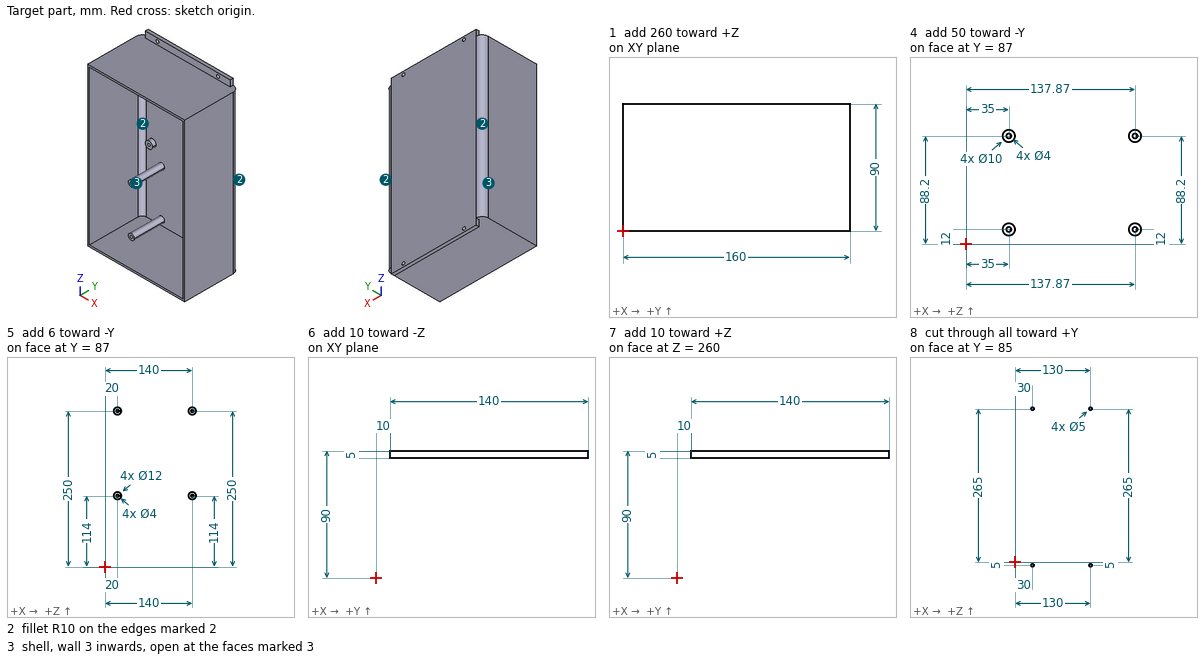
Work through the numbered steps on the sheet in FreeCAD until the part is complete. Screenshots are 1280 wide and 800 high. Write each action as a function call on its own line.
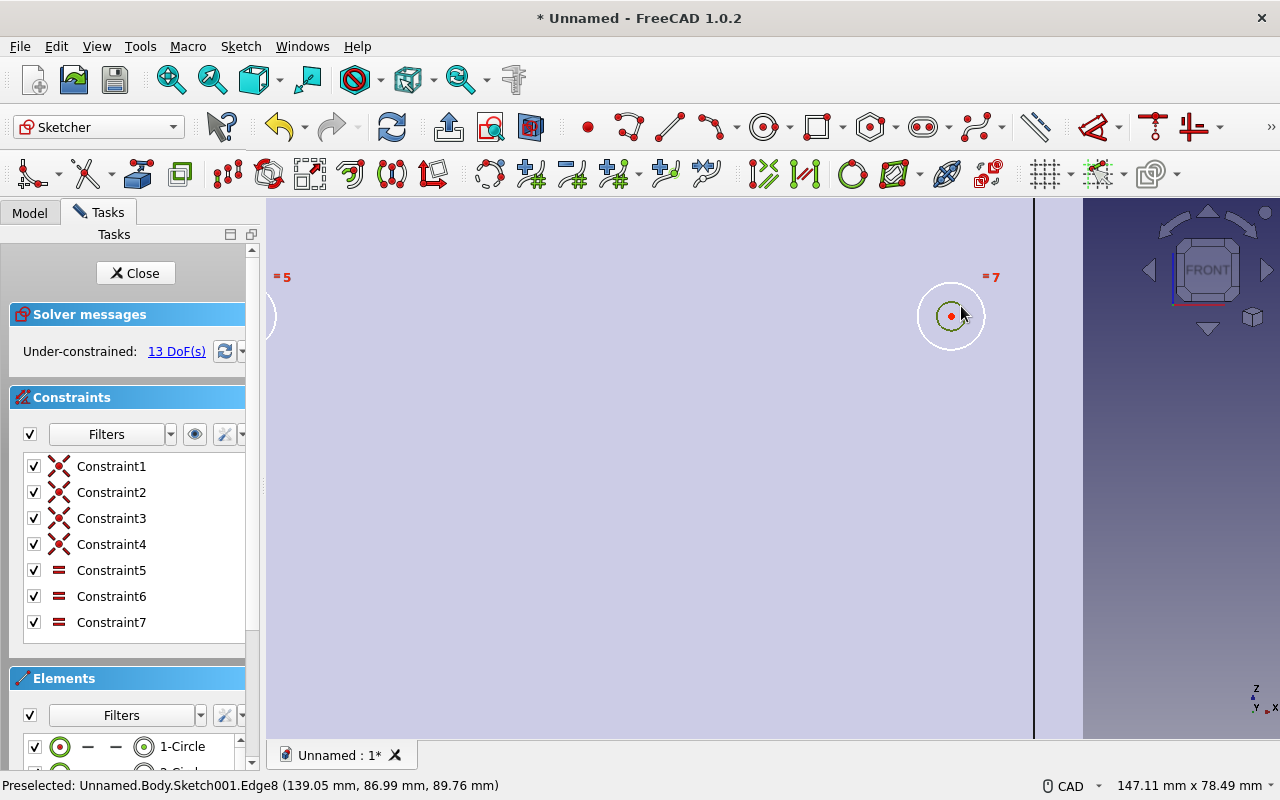
key(e)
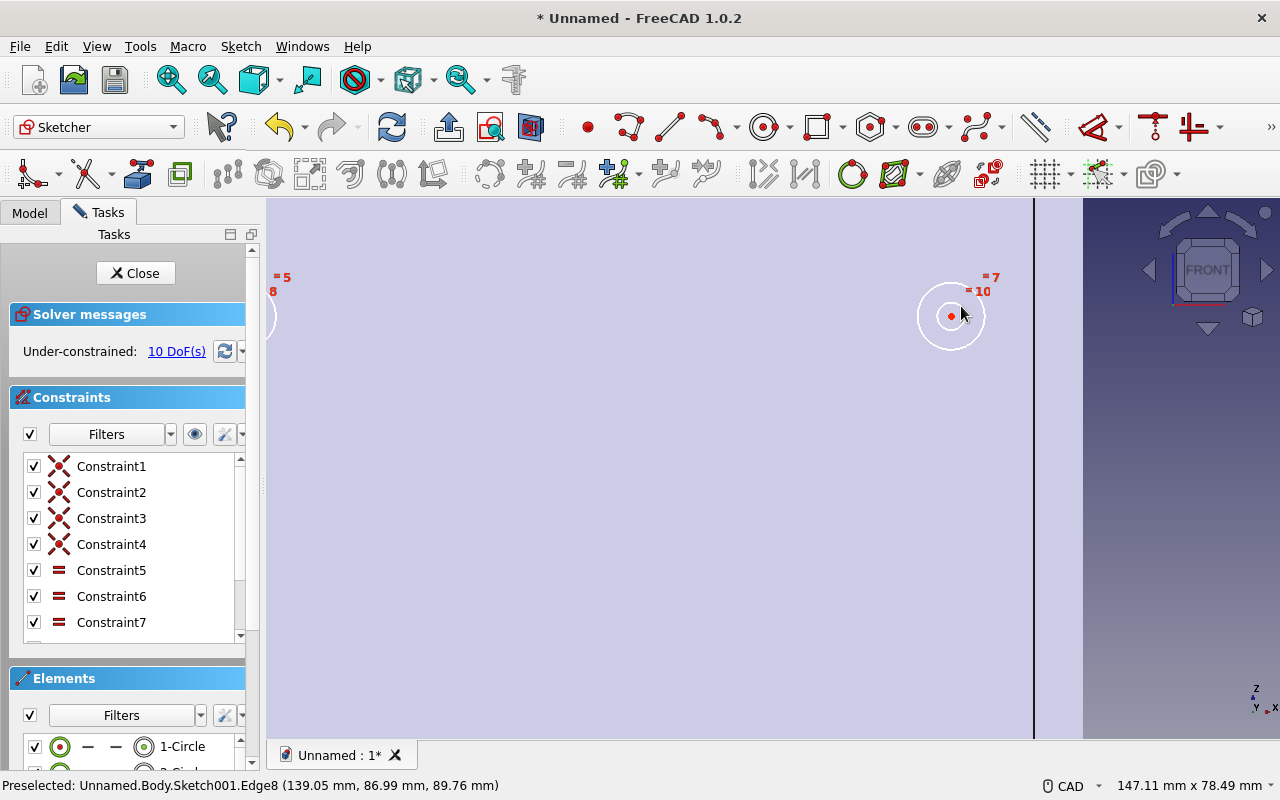
click(1092, 128)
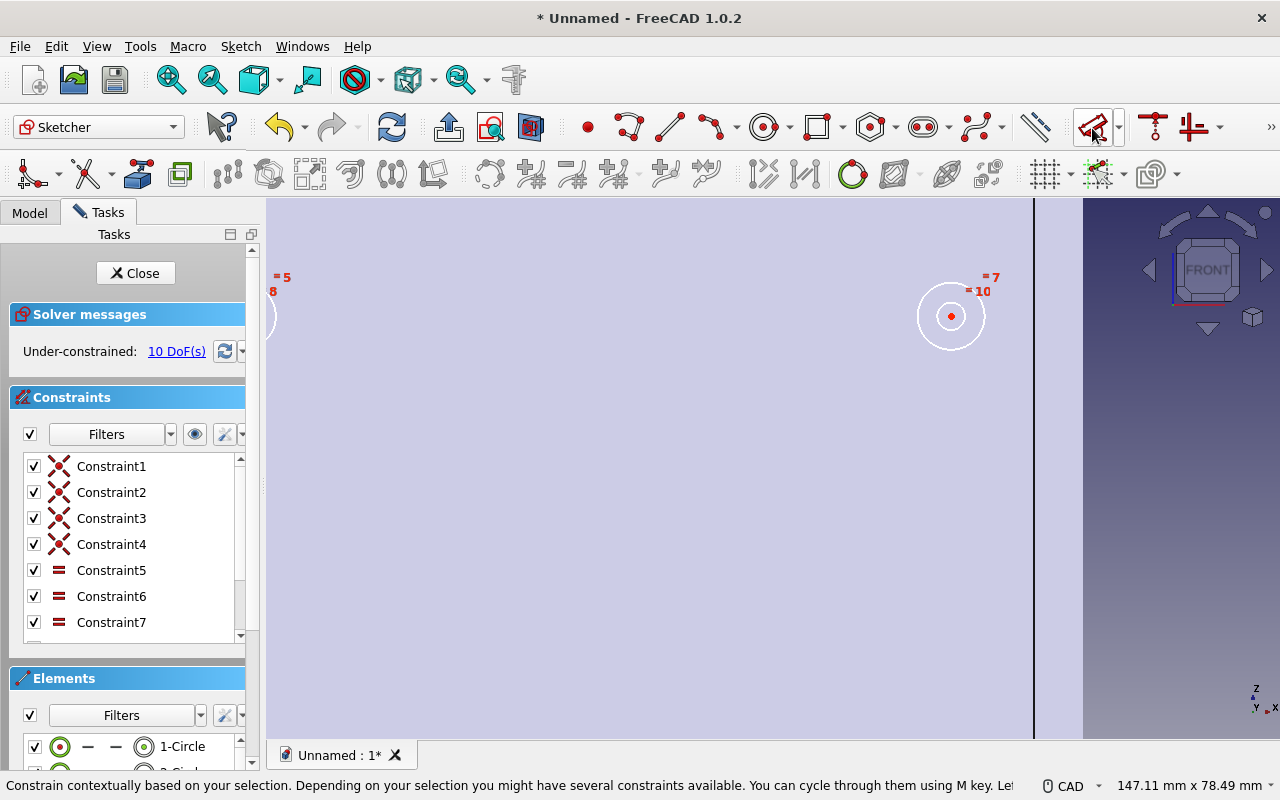
scroll(962, 306, down, 3)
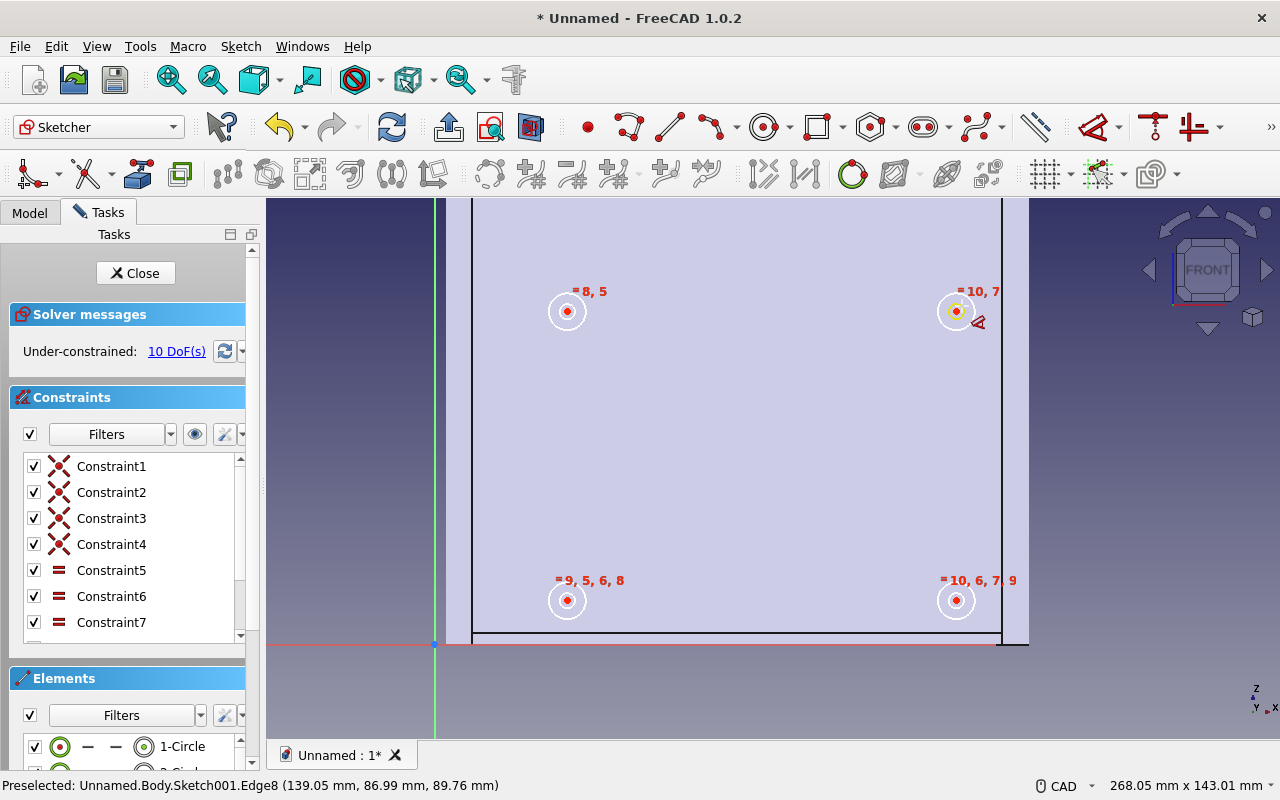
scroll(580, 299, up, 2)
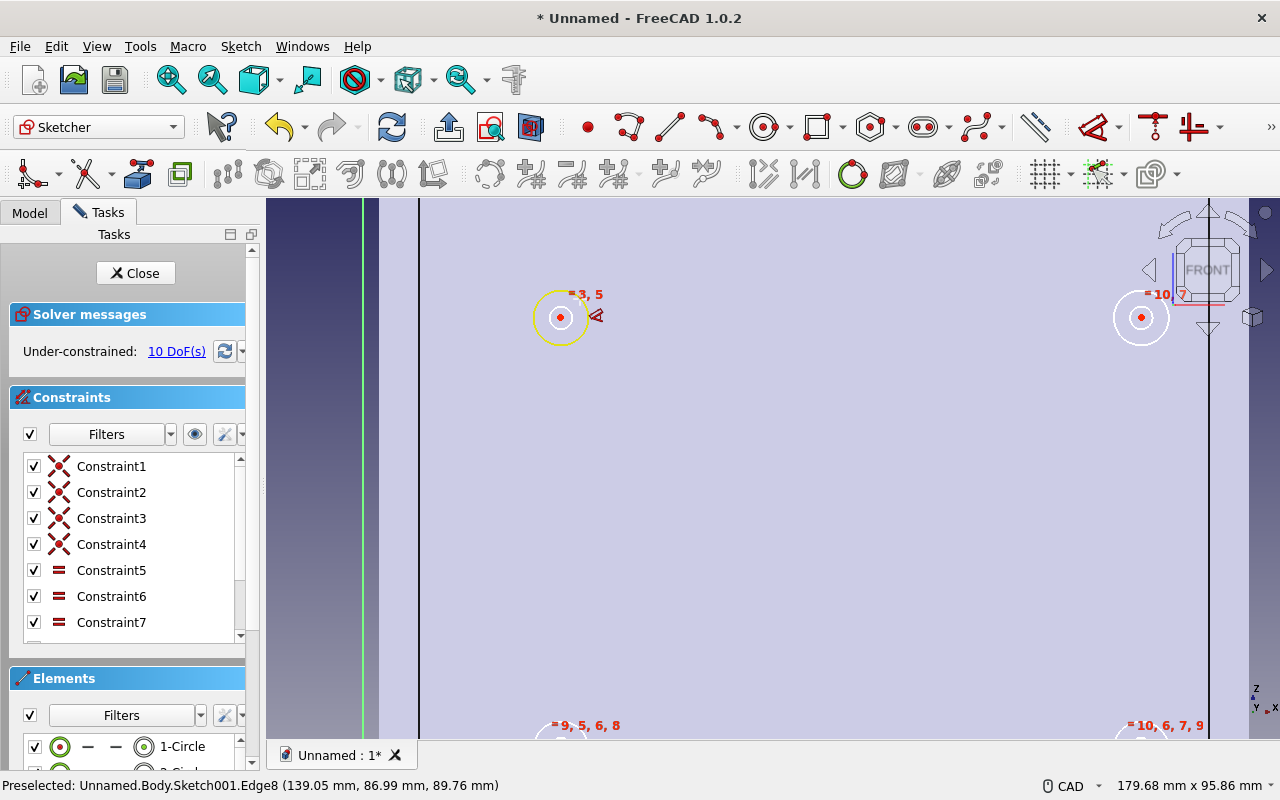
click(580, 298)
click(602, 275)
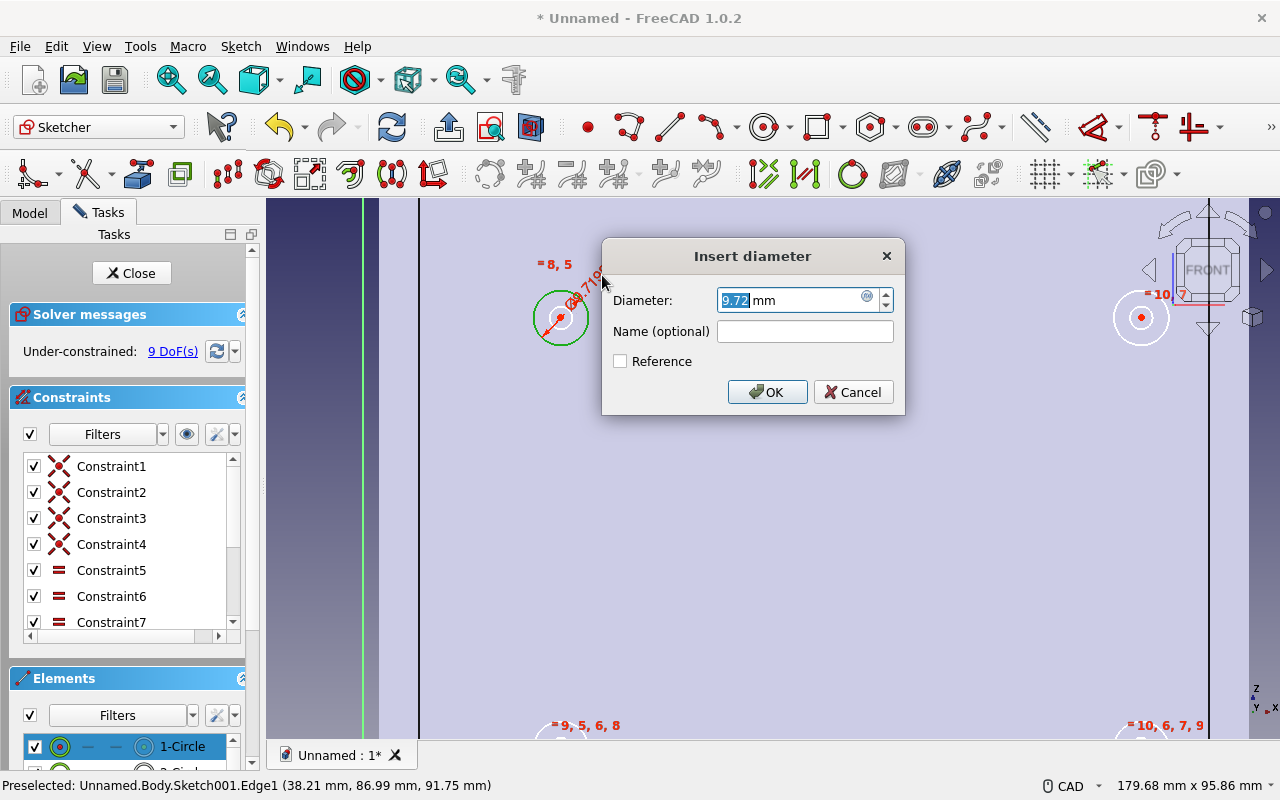
text(10)
key(Return)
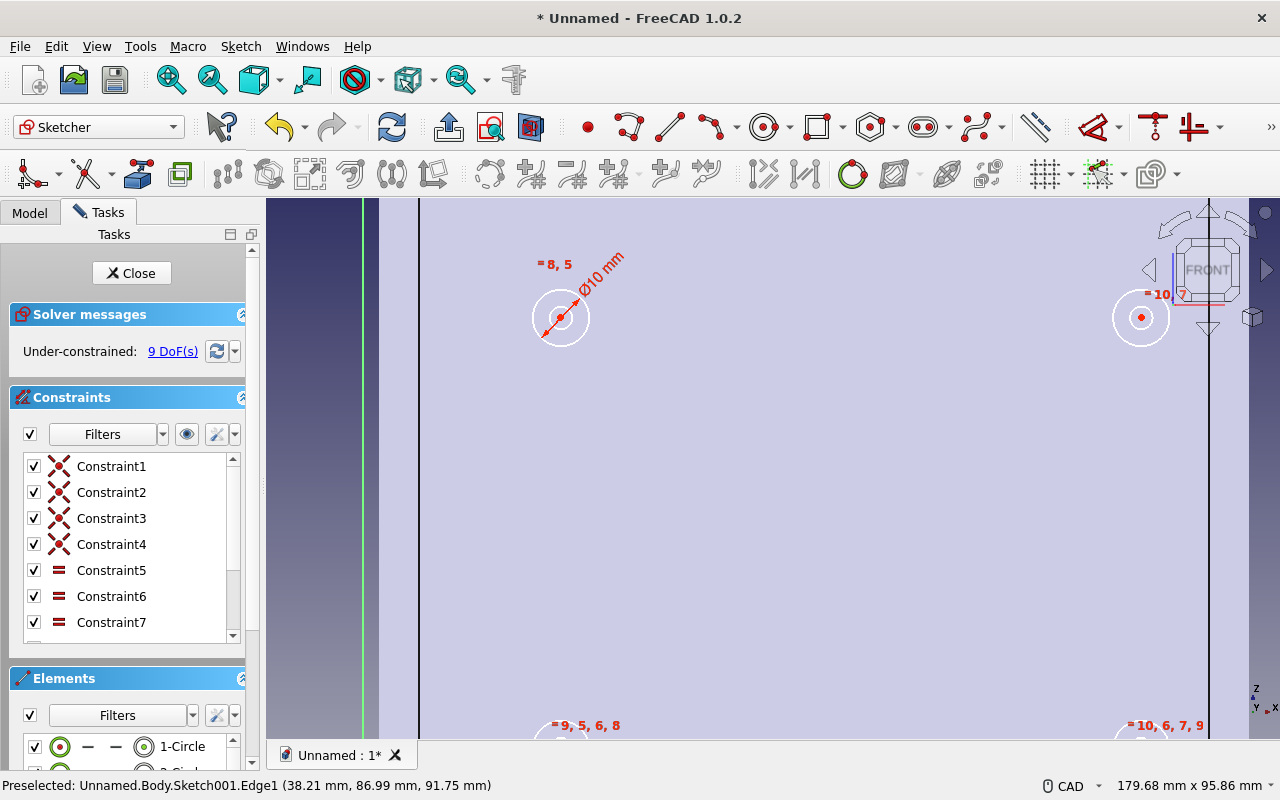
scroll(569, 310, up, 3)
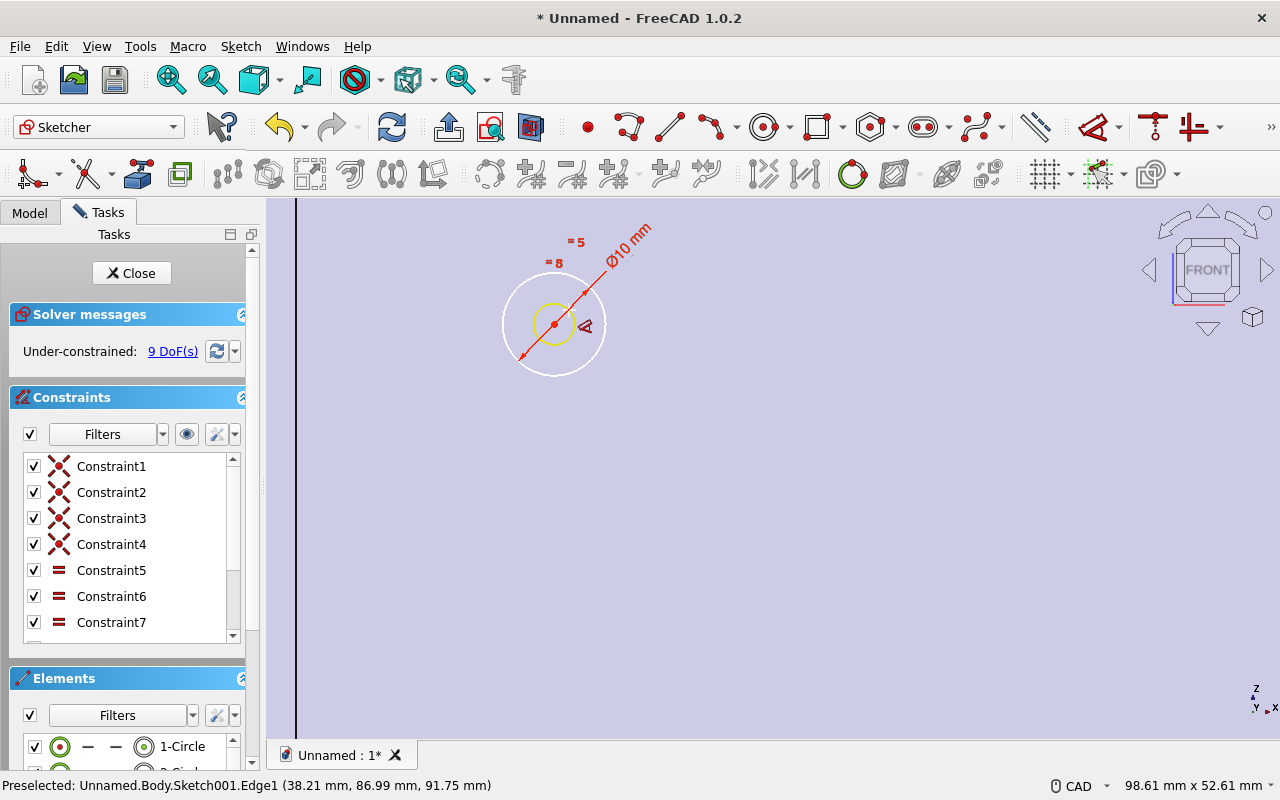
click(569, 310)
click(609, 272)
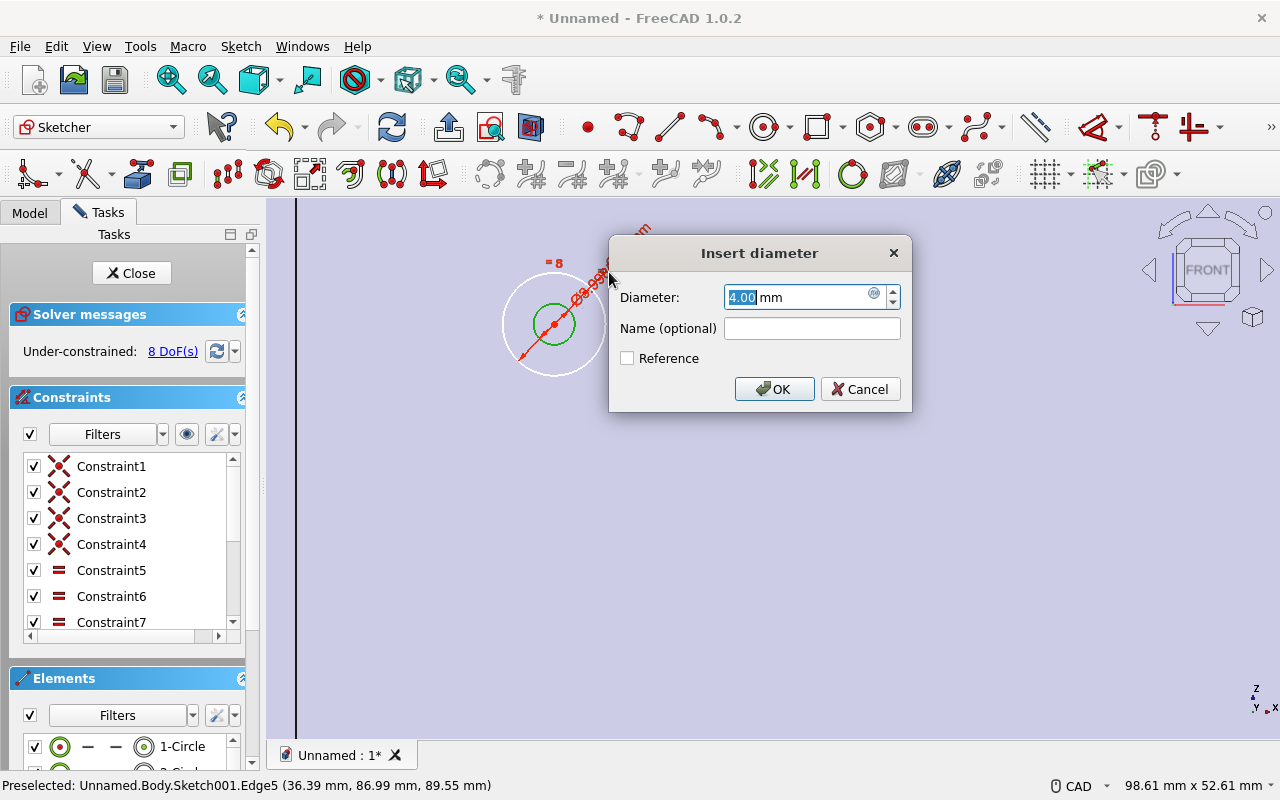
text(4)
key(Return)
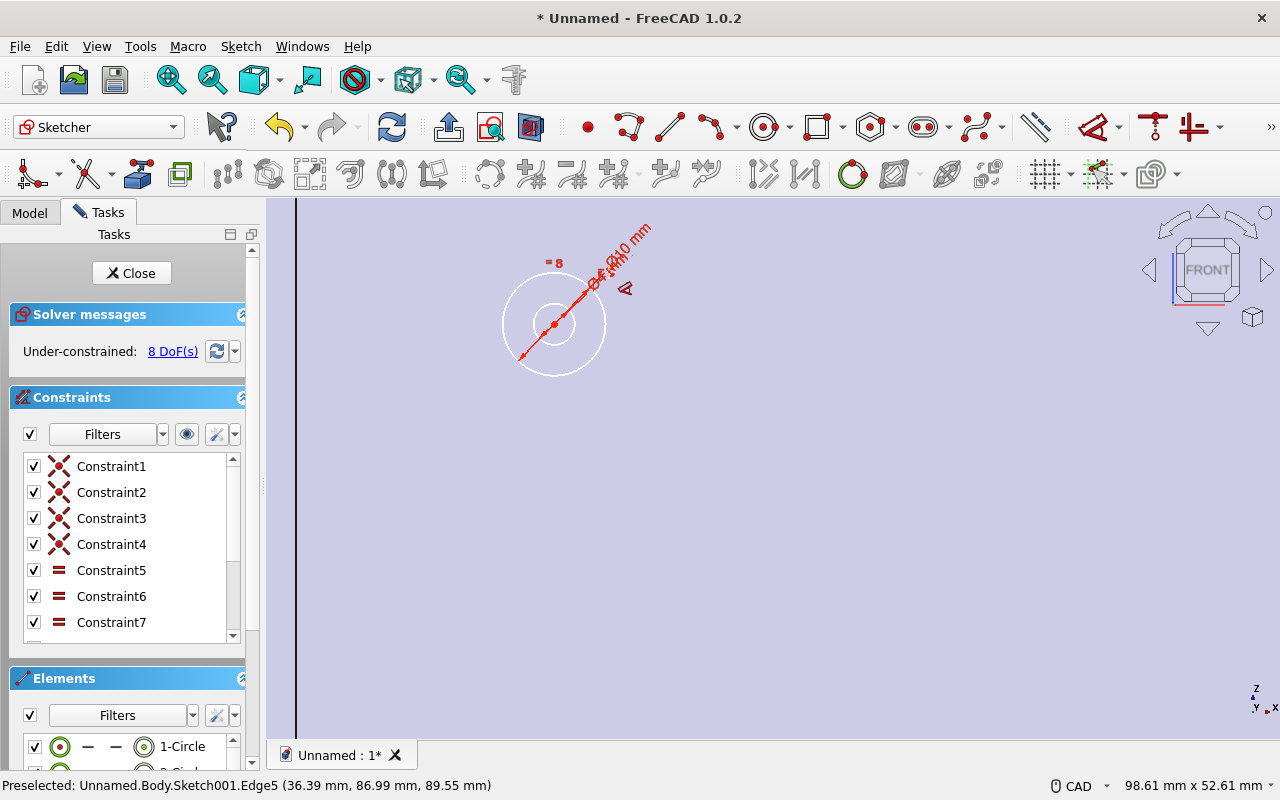
click(554, 324)
click(424, 290)